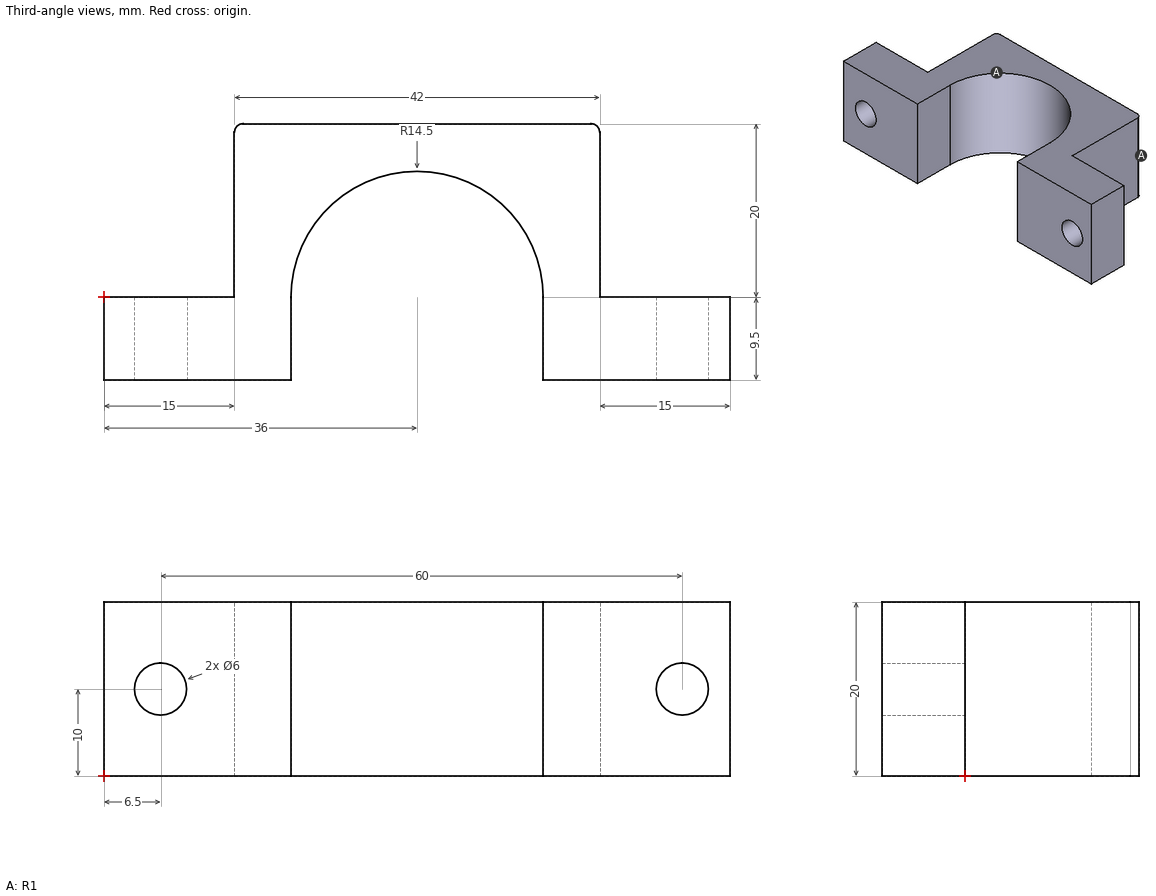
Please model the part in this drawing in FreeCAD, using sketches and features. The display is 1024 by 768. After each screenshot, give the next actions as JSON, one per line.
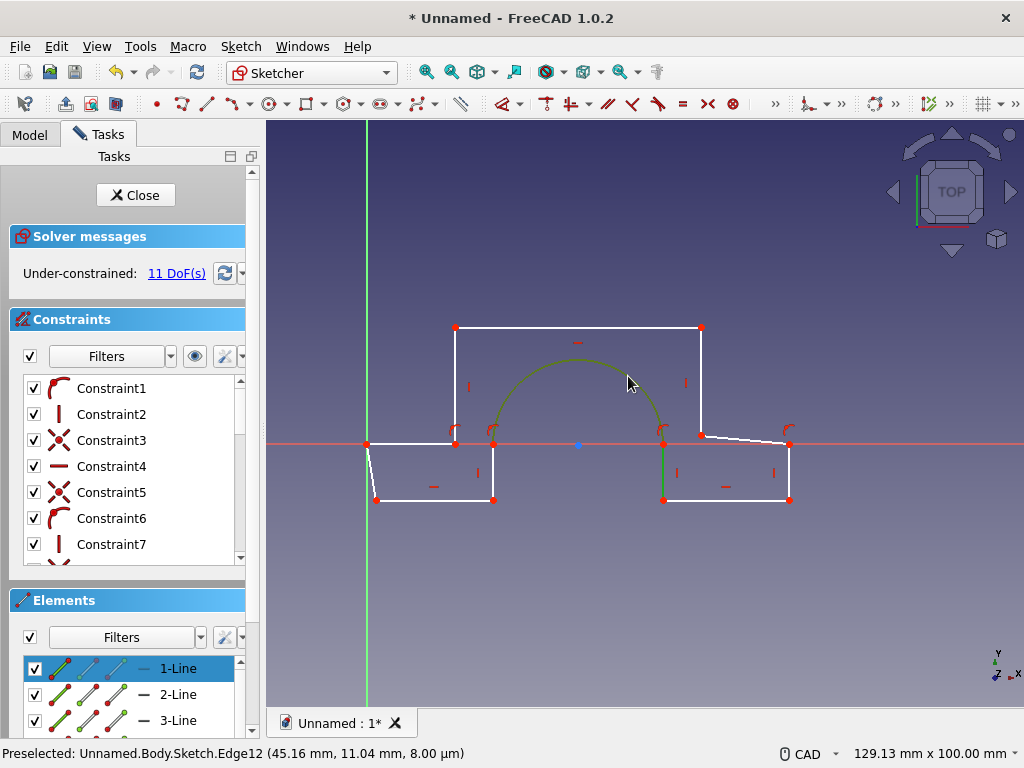
{"action": "left_click", "coordinate": [658, 104]}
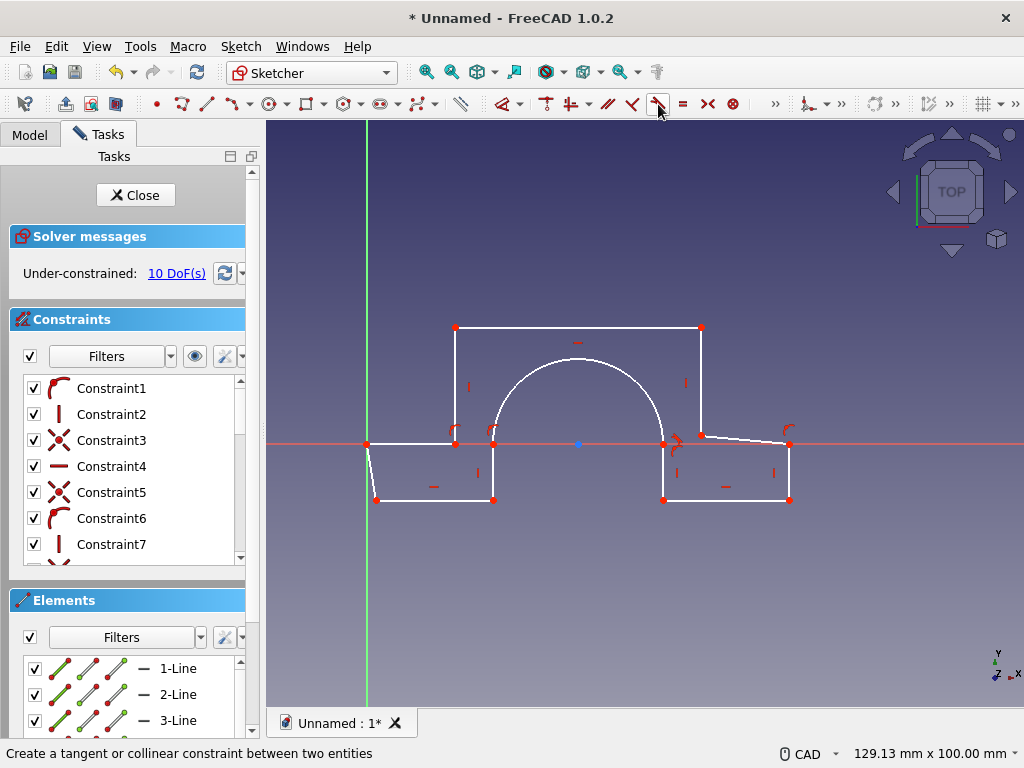
{"action": "left_click", "coordinate": [763, 442]}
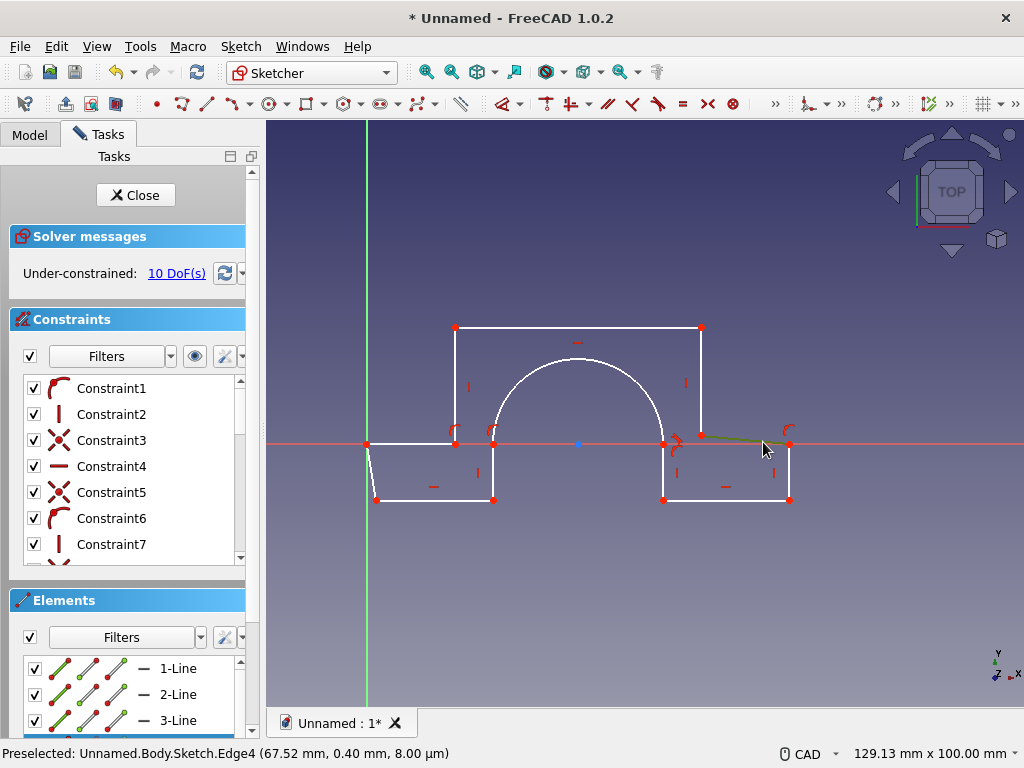
{"action": "left_click", "coordinate": [588, 104]}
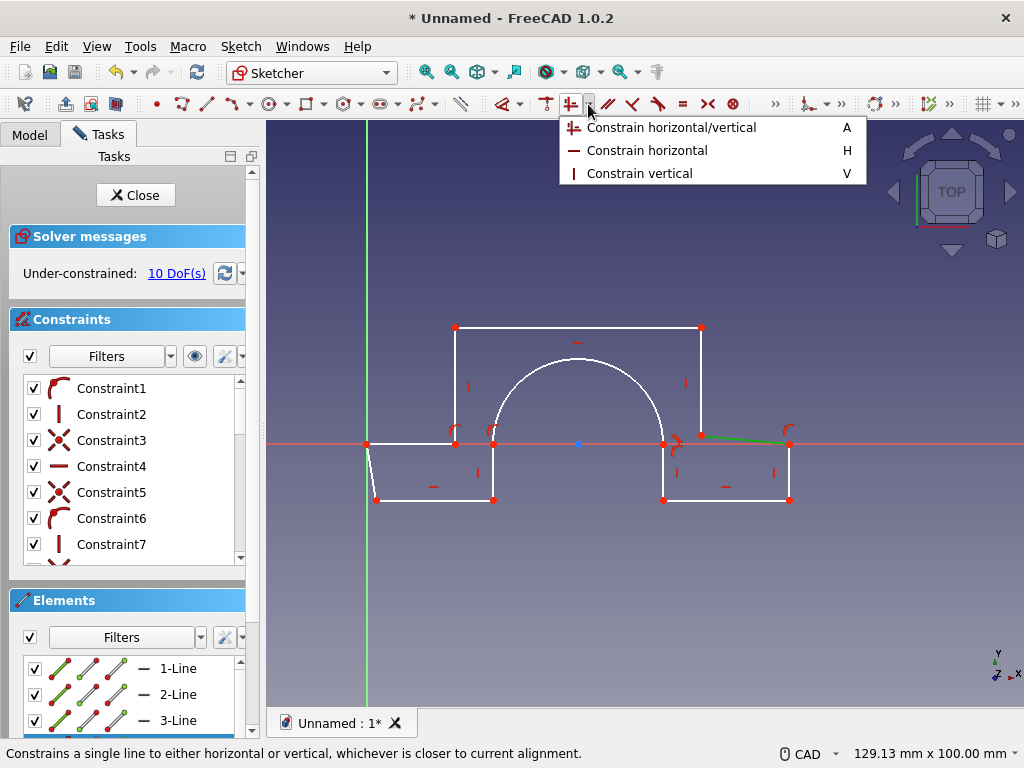
{"action": "left_click", "coordinate": [713, 150]}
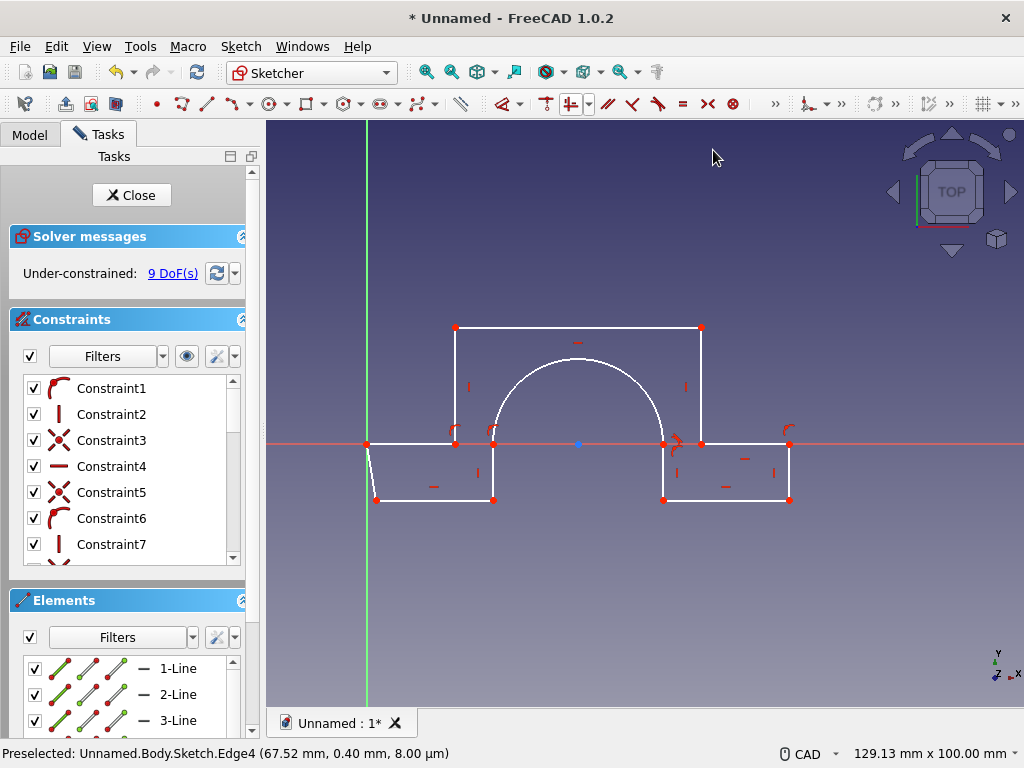
{"action": "left_click", "coordinate": [370, 461]}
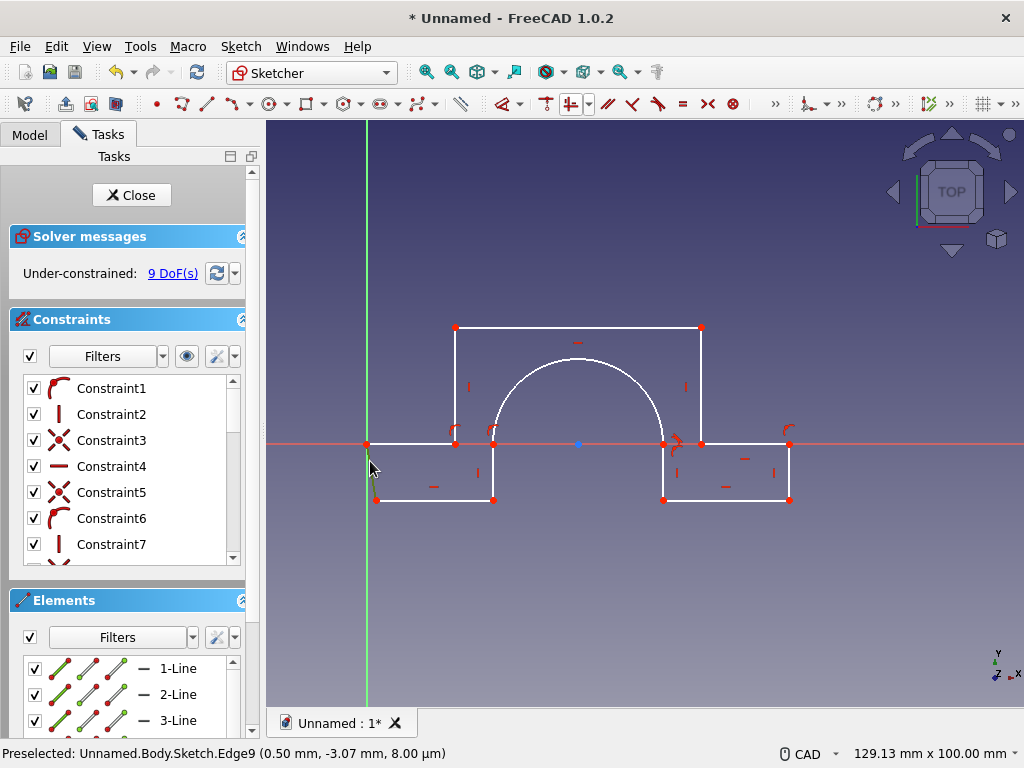
{"action": "key", "text": "v"}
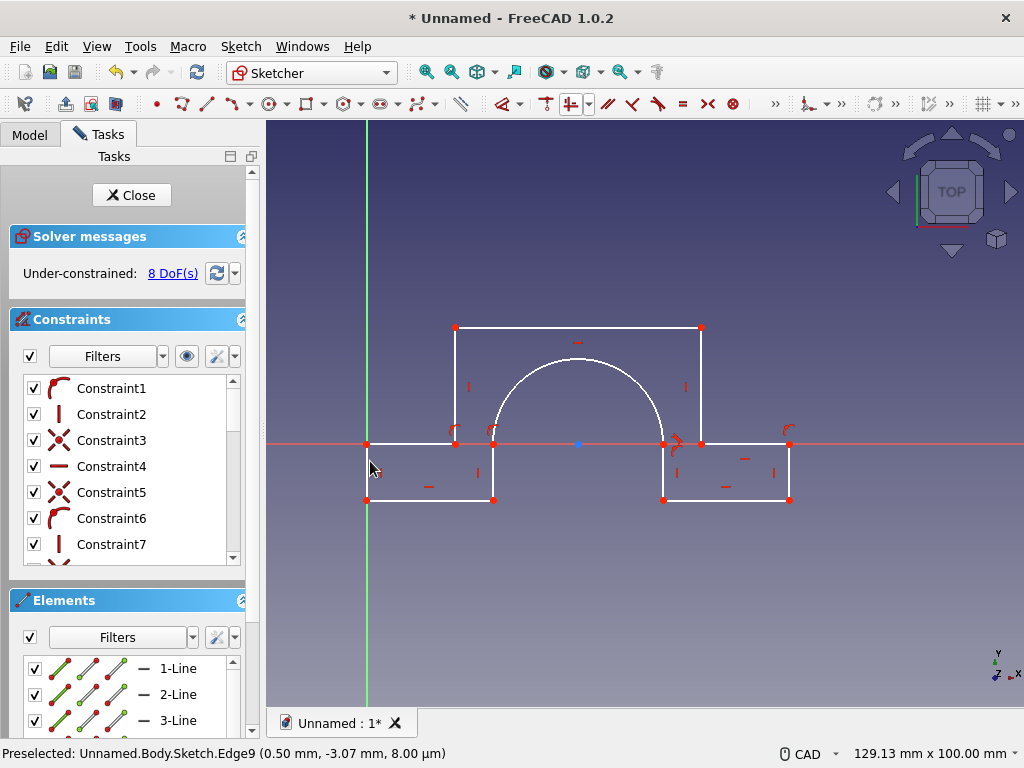
{"action": "left_click", "coordinate": [502, 104]}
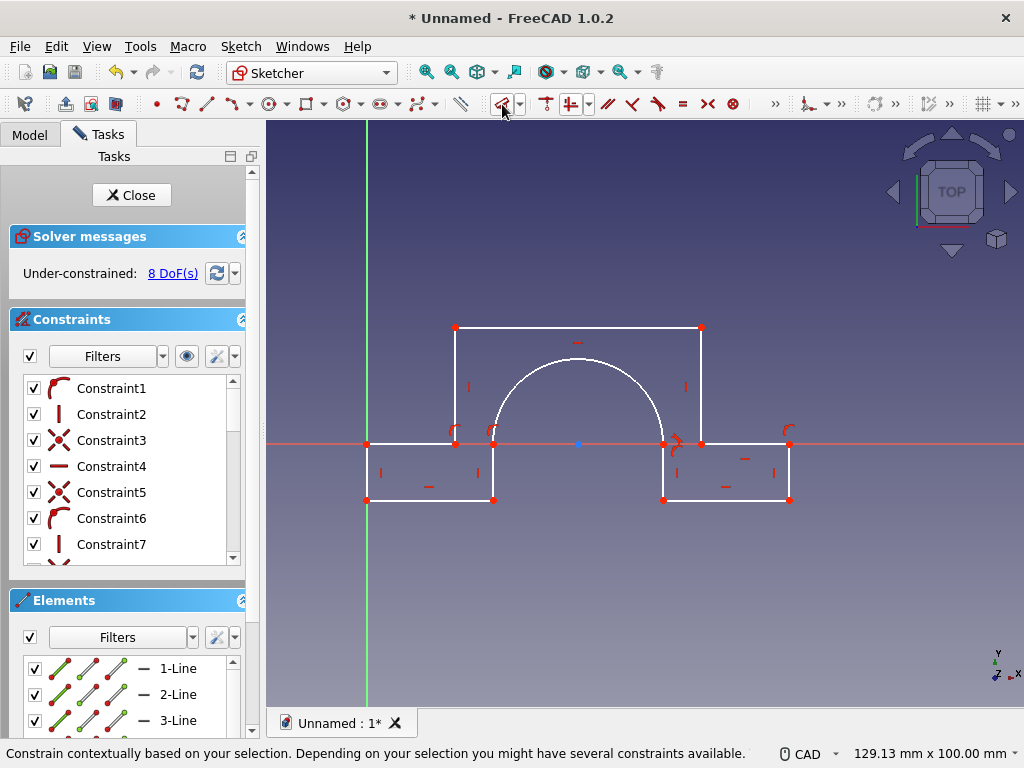
{"action": "left_click", "coordinate": [628, 375]}
{"action": "left_click", "coordinate": [647, 349]}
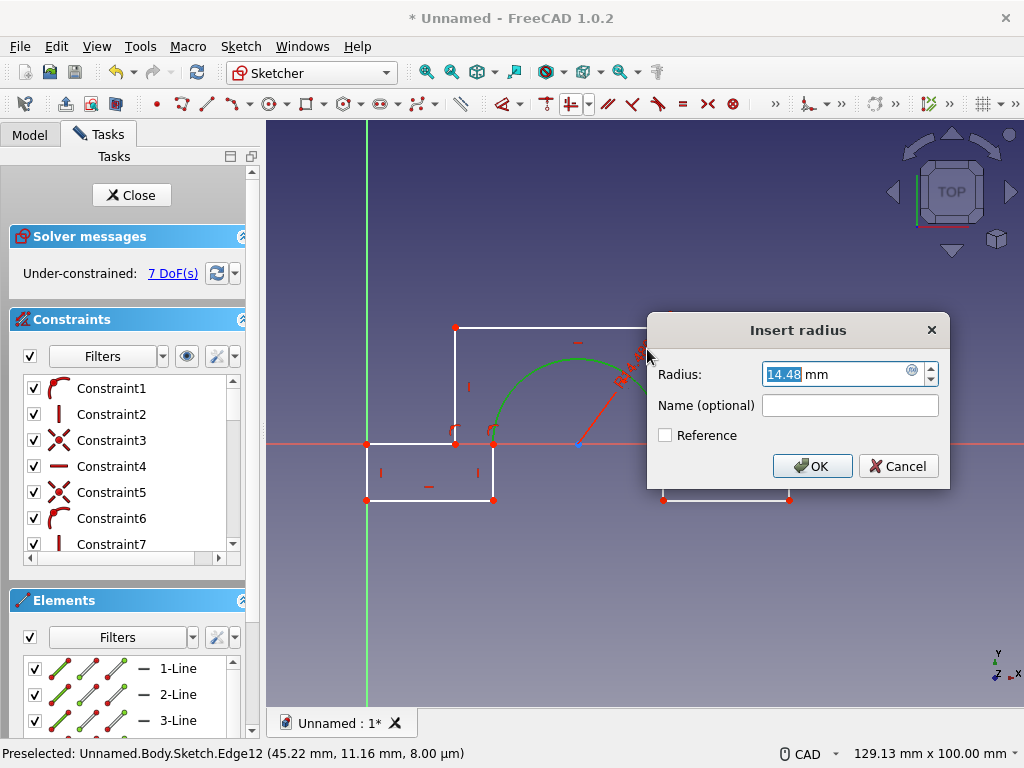
{"action": "type", "text": "14.5"}
{"action": "key", "text": "Return"}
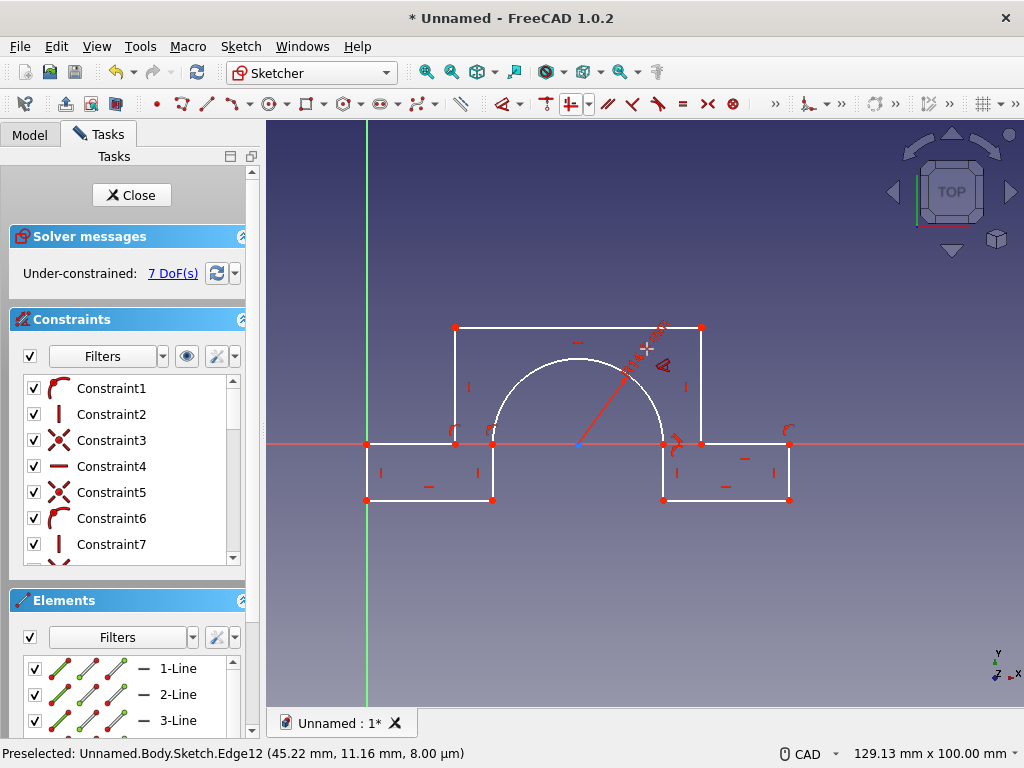
{"action": "left_click", "coordinate": [763, 444]}
{"action": "left_click", "coordinate": [745, 478]}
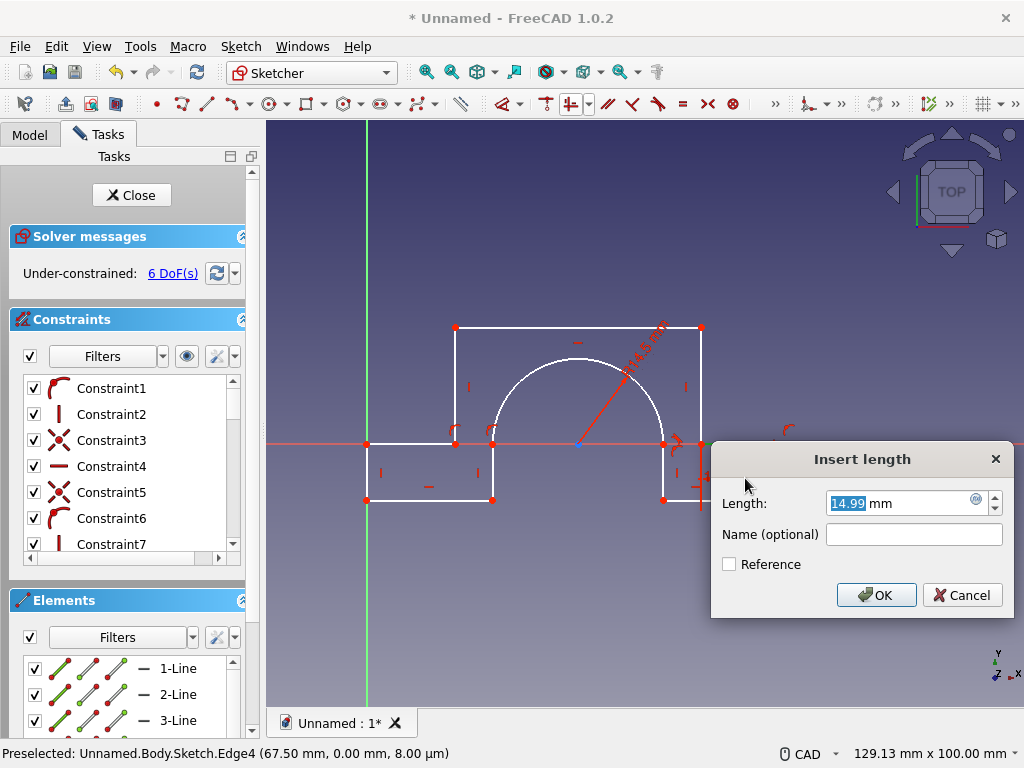
{"action": "type", "text": "15"}
{"action": "key", "text": "Return"}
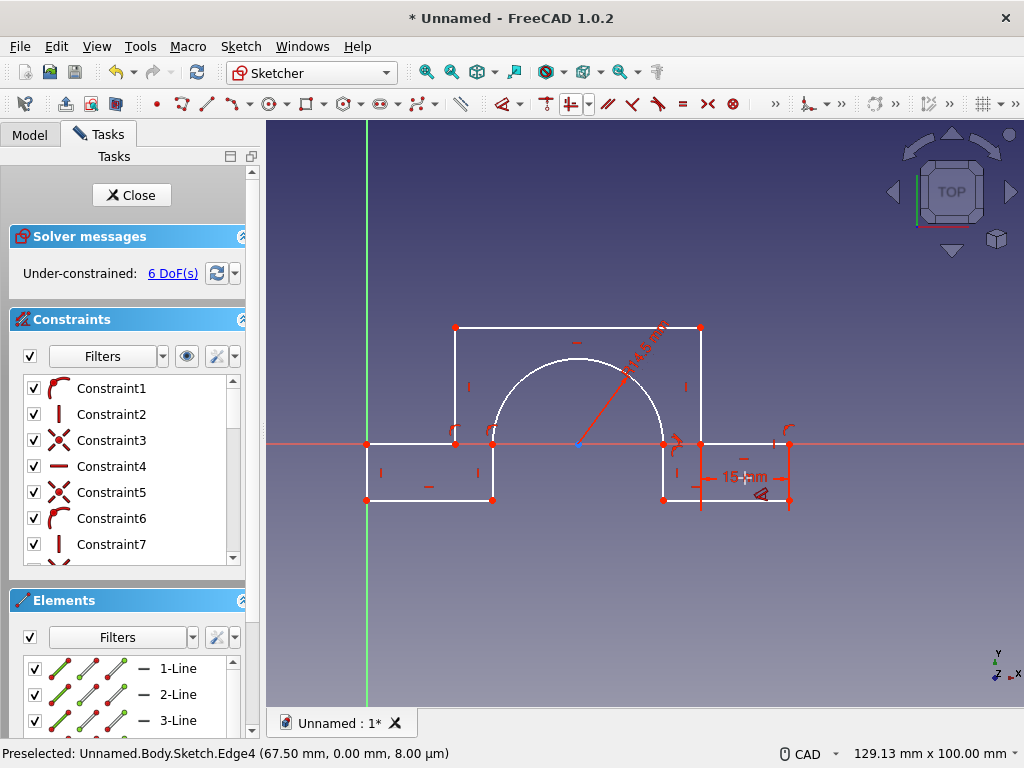
{"action": "left_click", "coordinate": [701, 409]}
{"action": "left_click", "coordinate": [735, 386]}